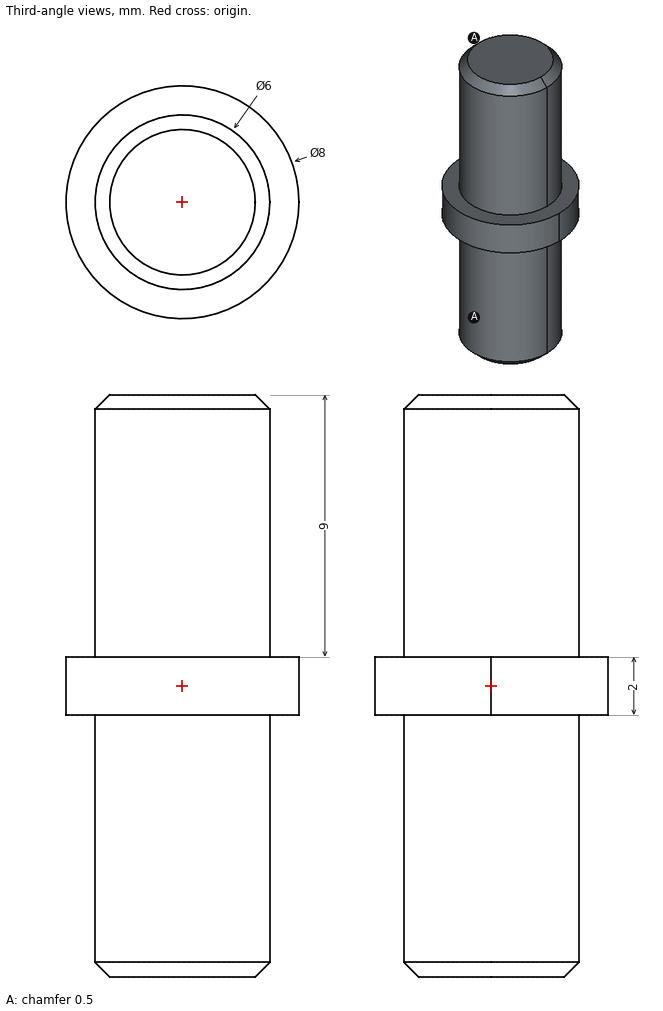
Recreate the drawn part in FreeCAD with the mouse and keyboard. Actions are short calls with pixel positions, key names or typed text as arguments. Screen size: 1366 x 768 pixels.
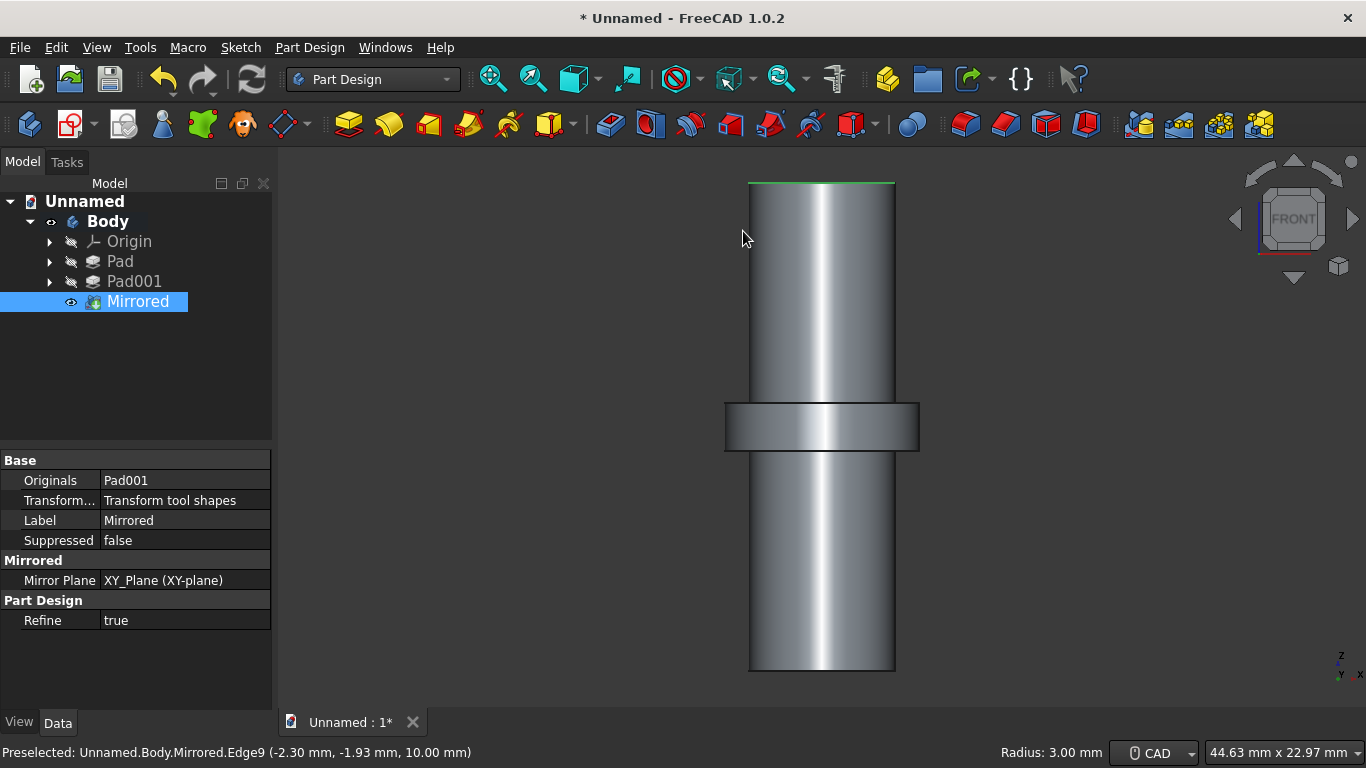
click(763, 670, ctrl)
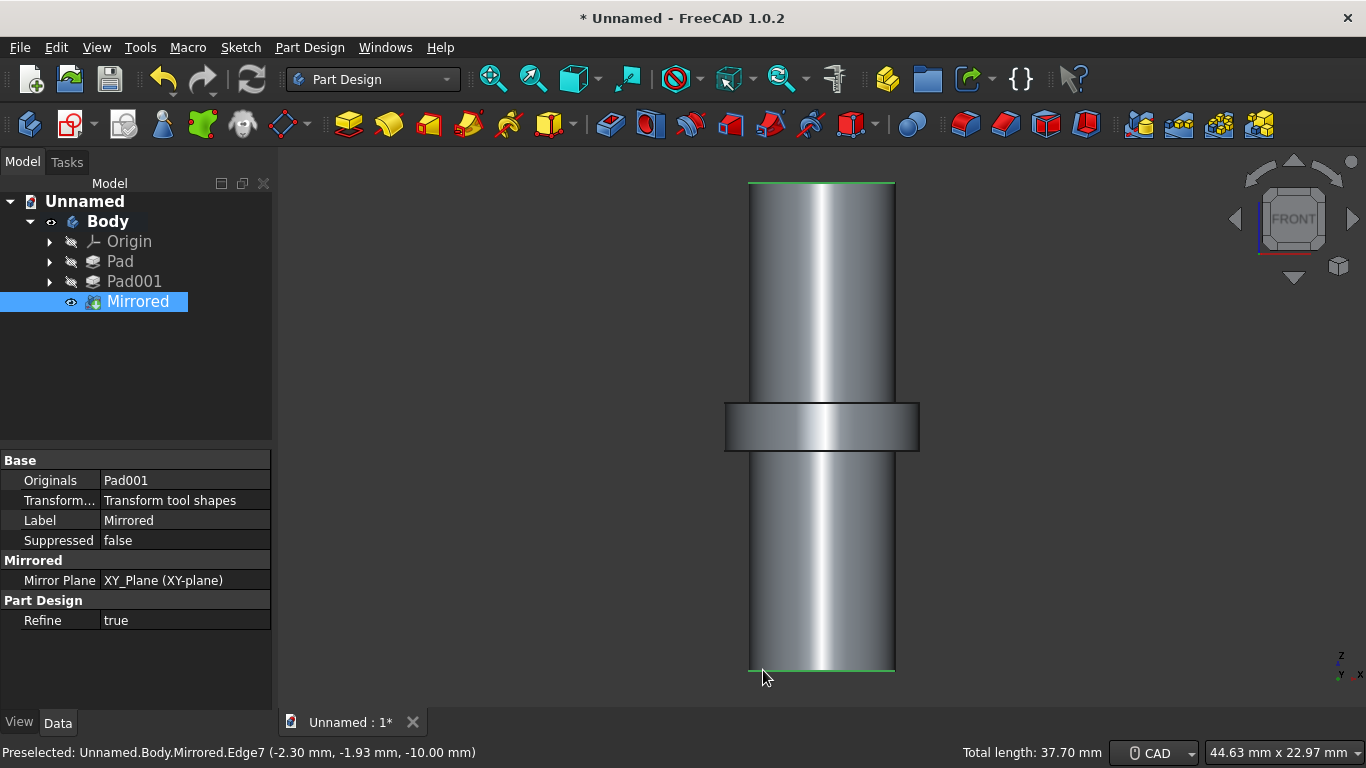
click(1006, 124)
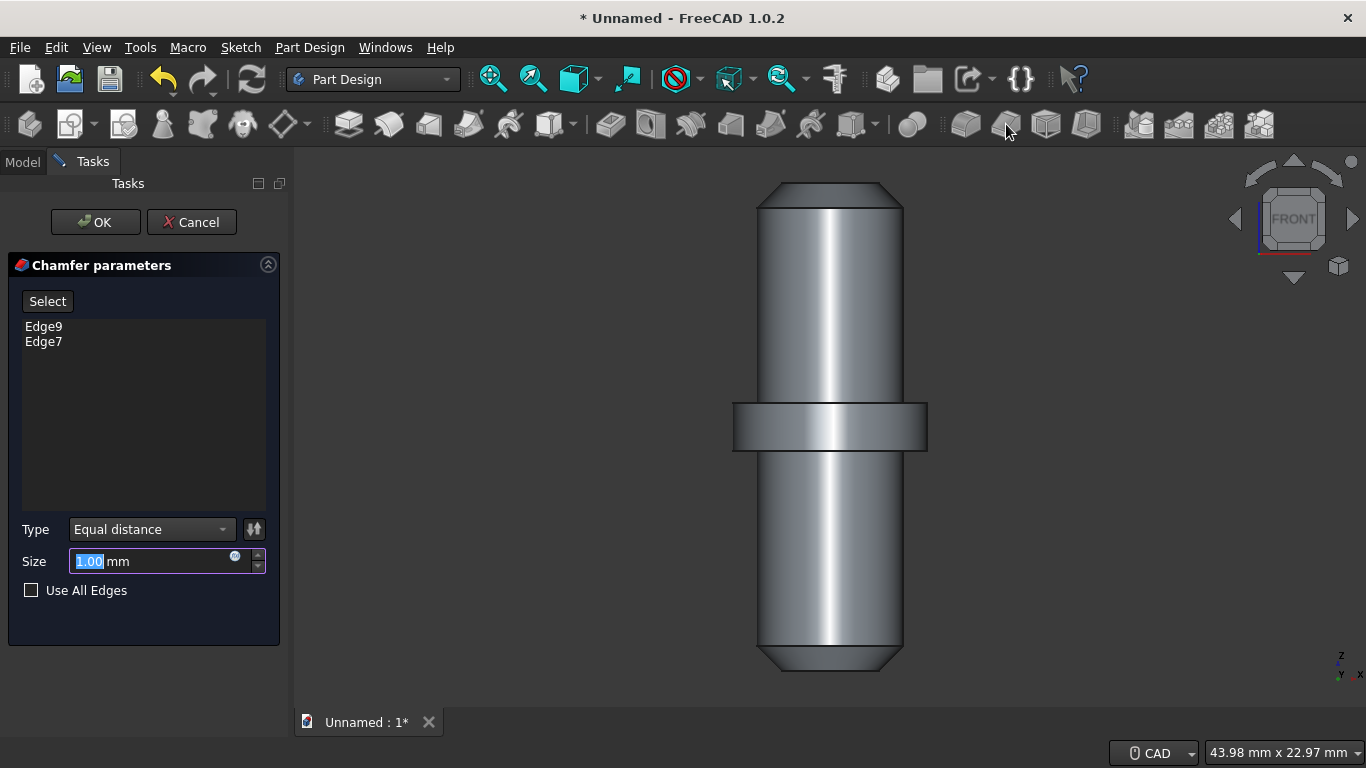
text(0.5)
key(Tab)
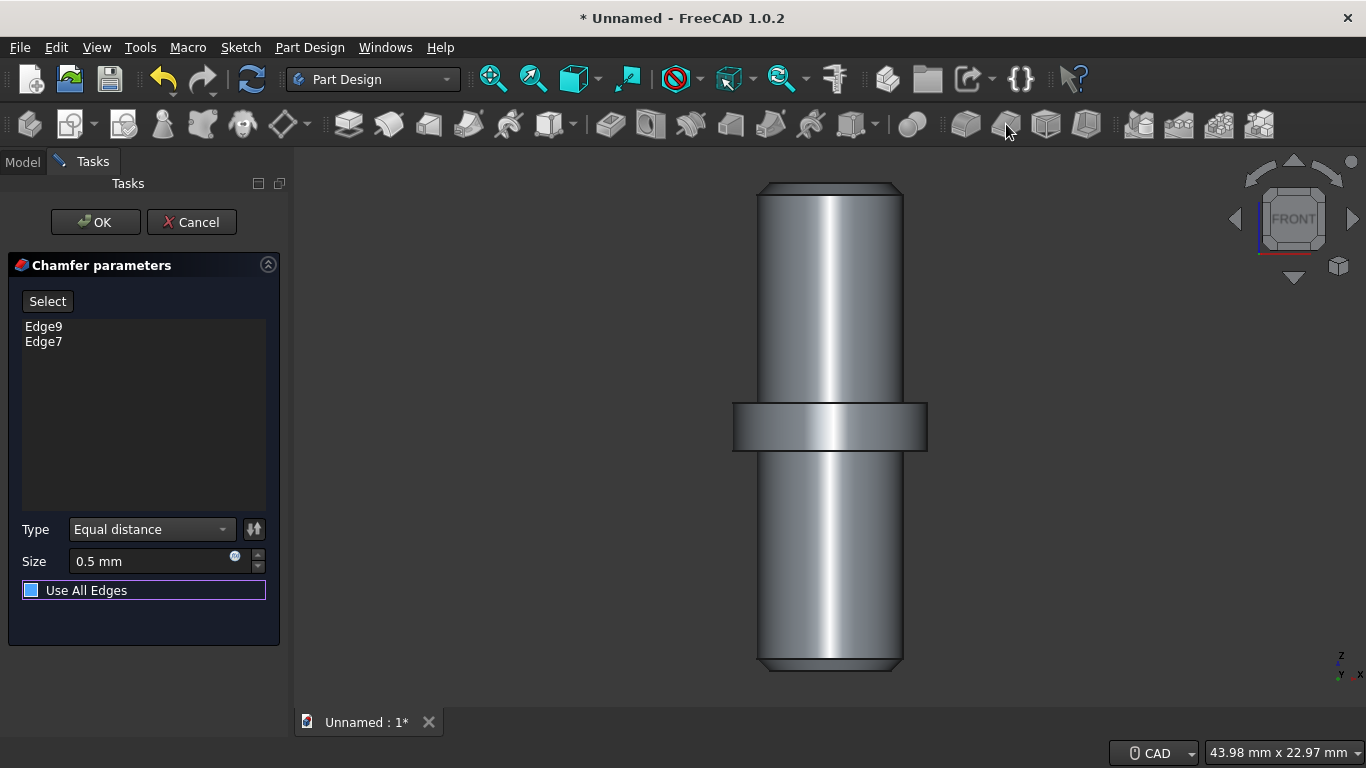
click(96, 222)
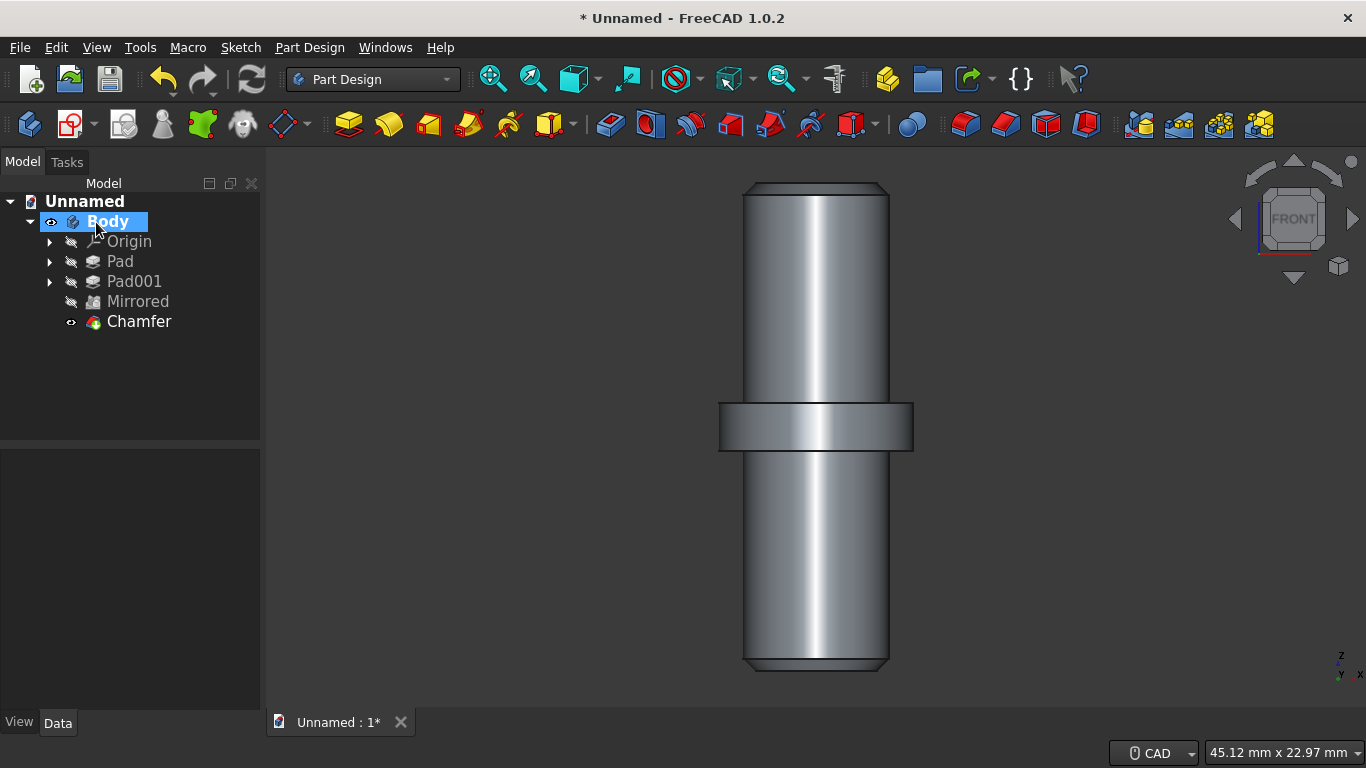
key(0)